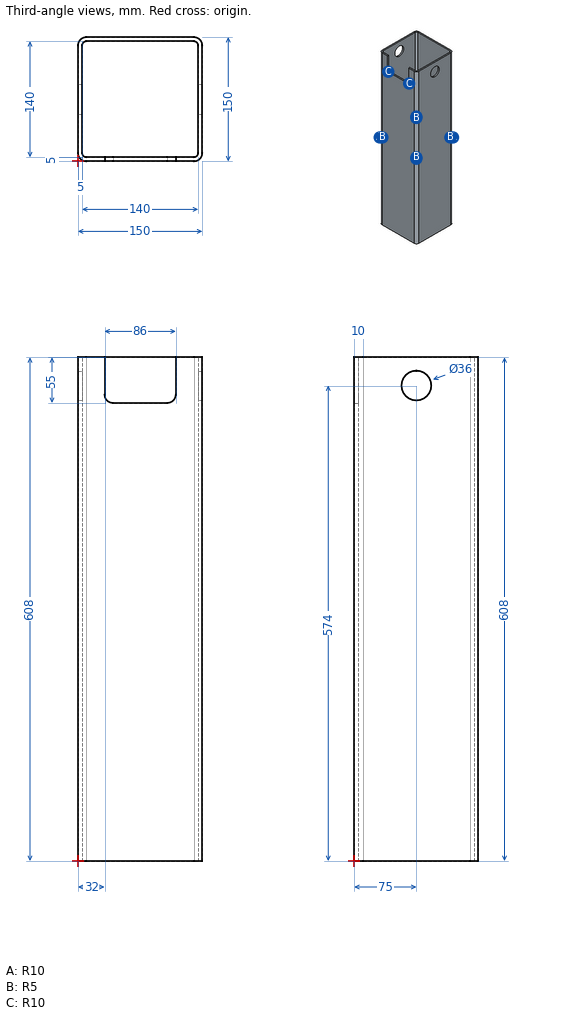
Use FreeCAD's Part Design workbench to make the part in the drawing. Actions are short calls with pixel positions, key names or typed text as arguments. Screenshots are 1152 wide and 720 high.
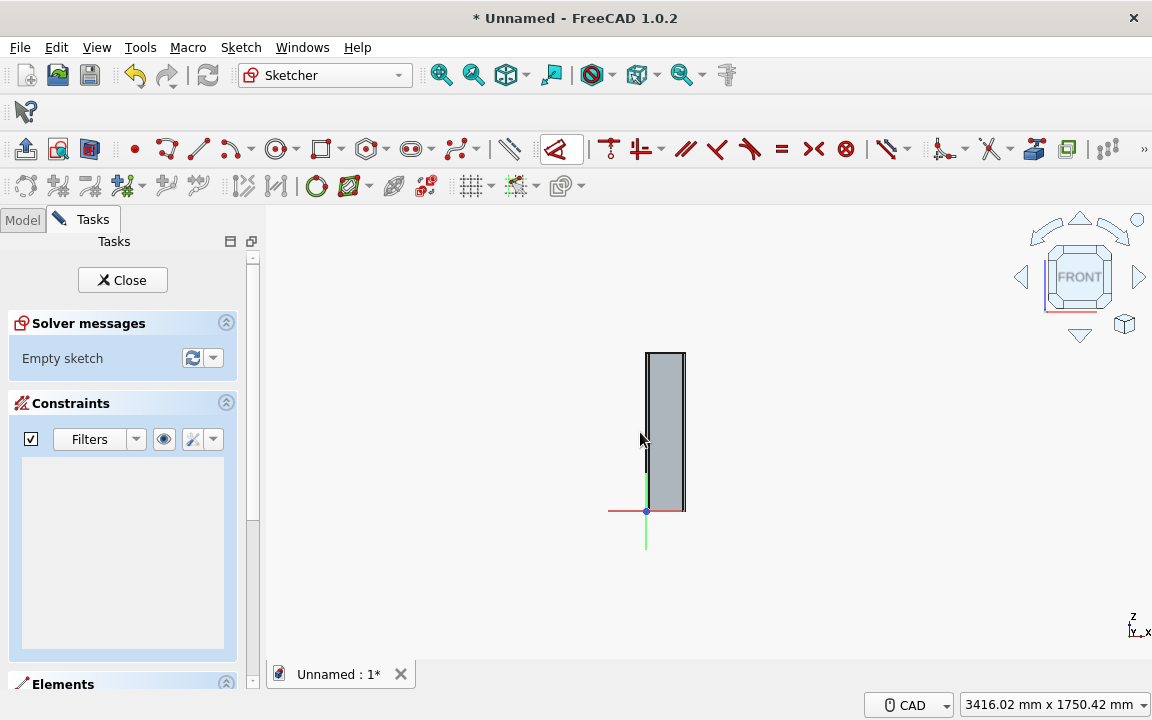
scroll(667, 357, up, 15)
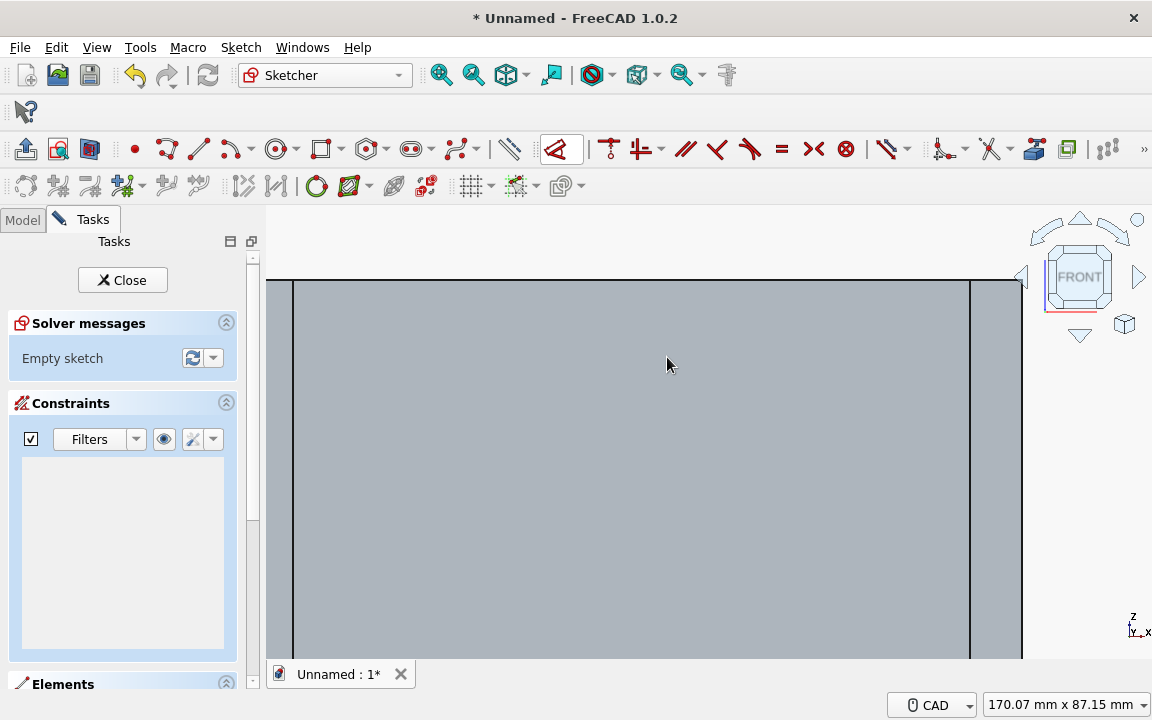
key(g)
key(r)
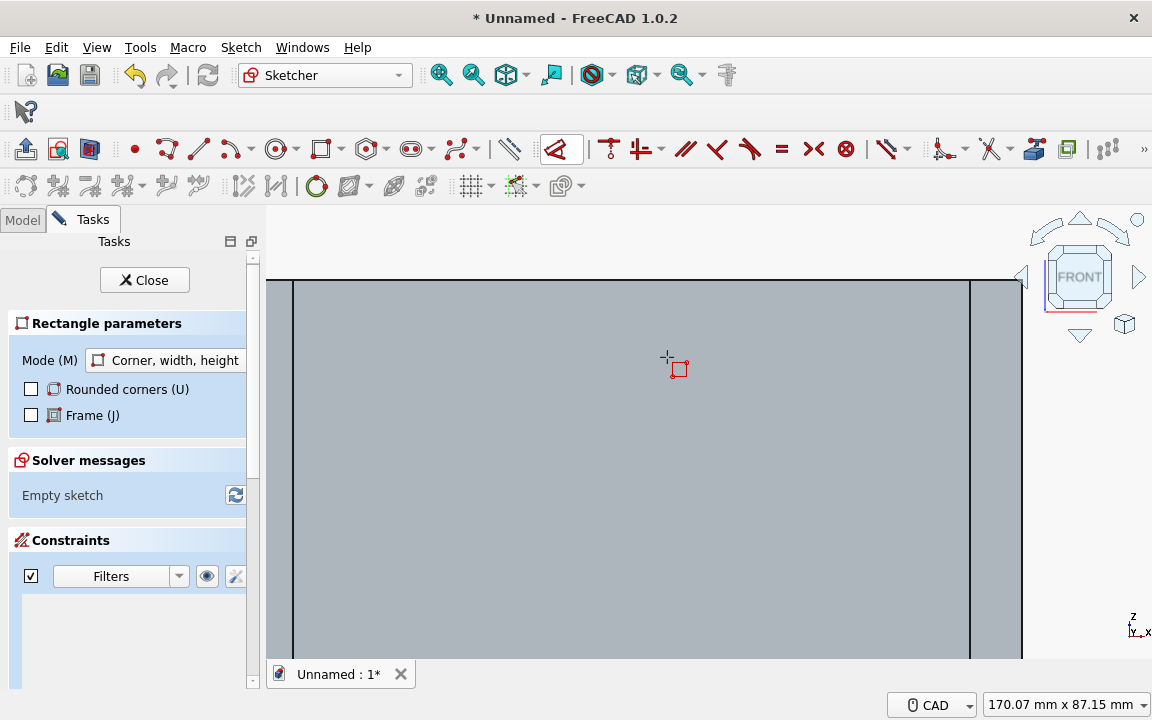
click(407, 280)
click(855, 566)
key(Escape)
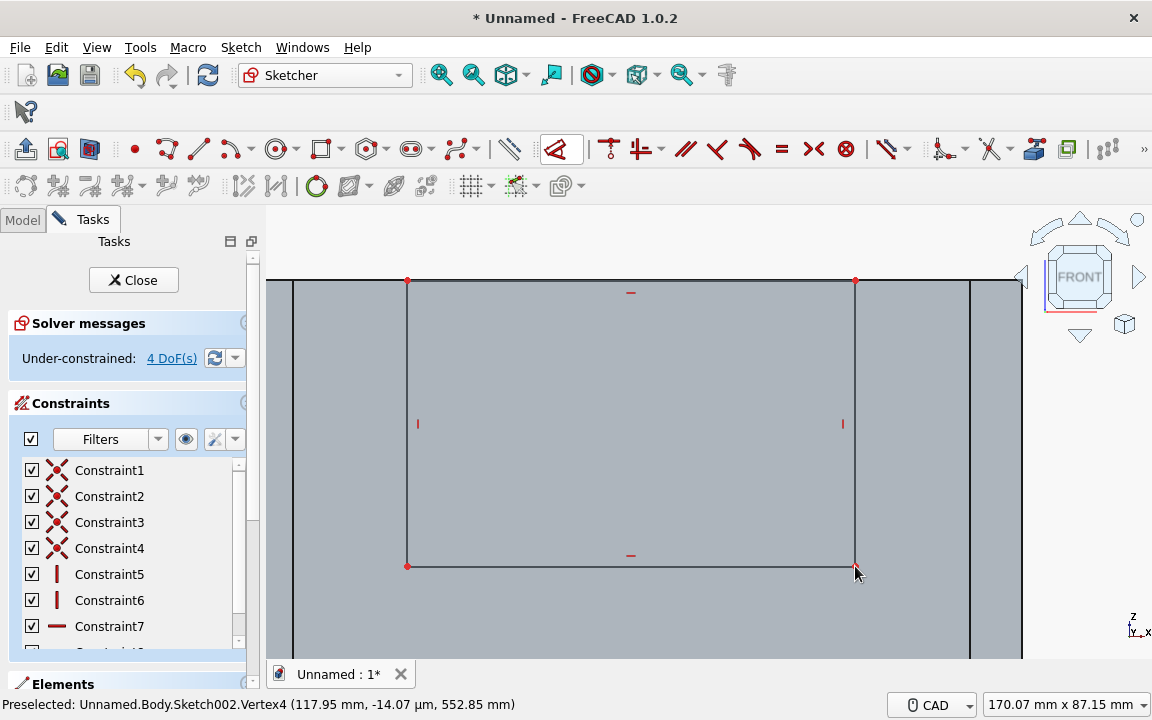
click(407, 367)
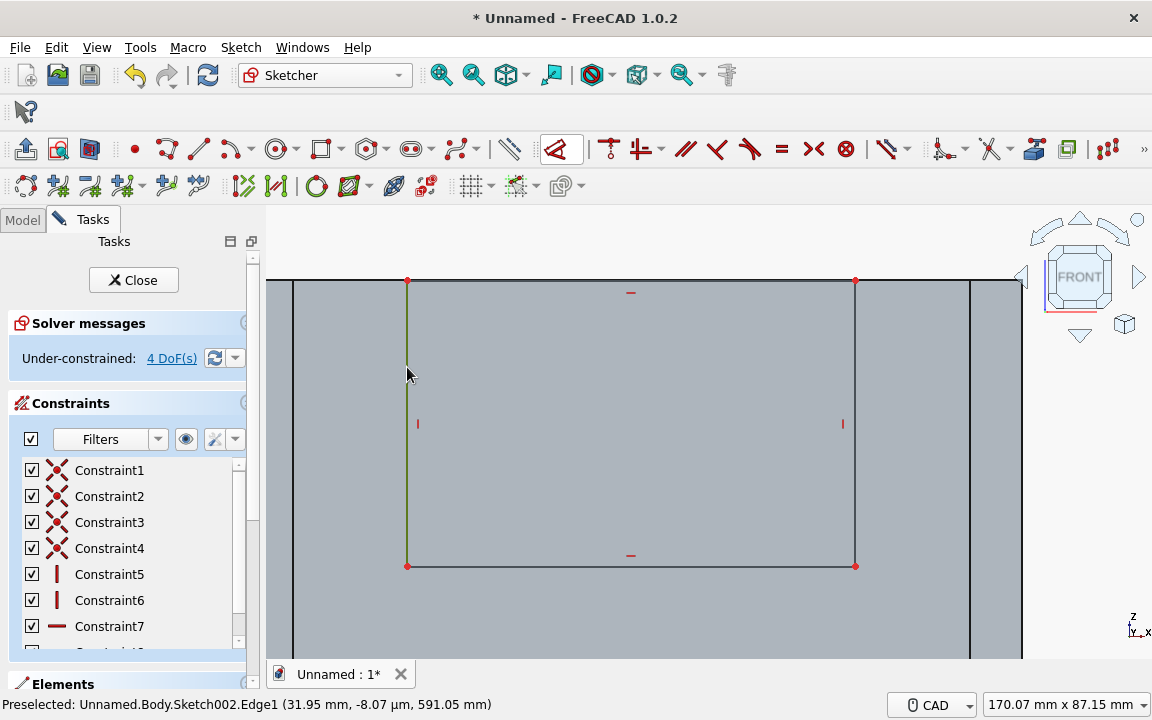
key(i)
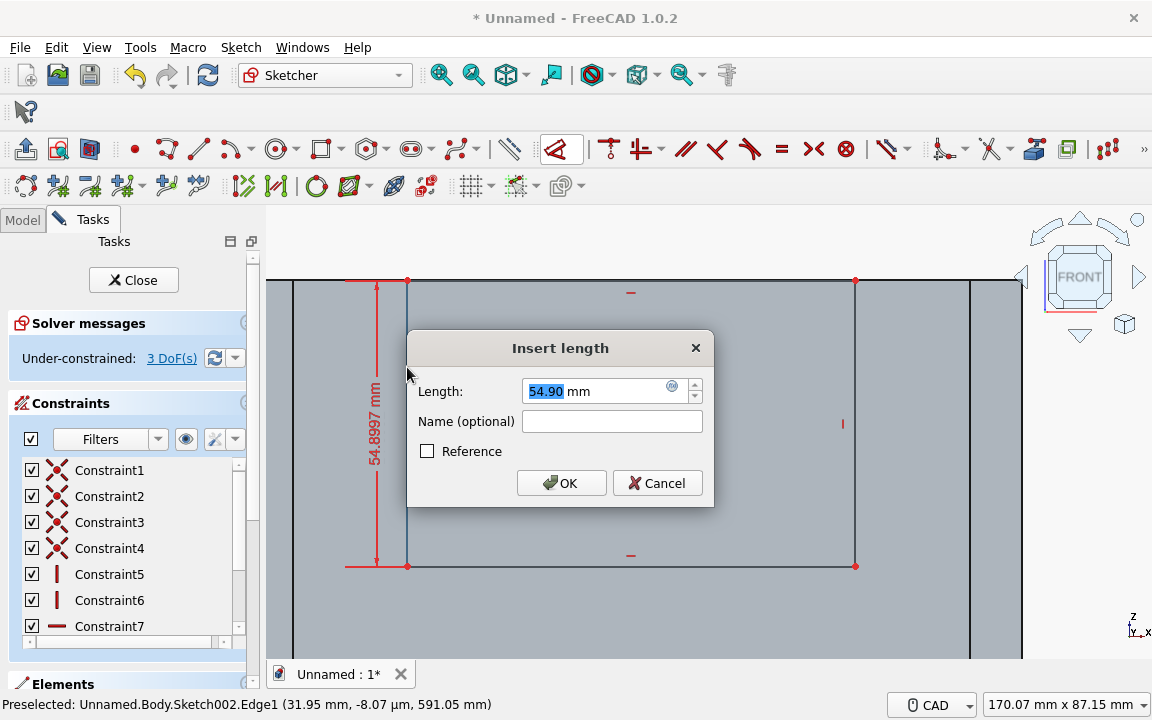
text(55)
key(Return)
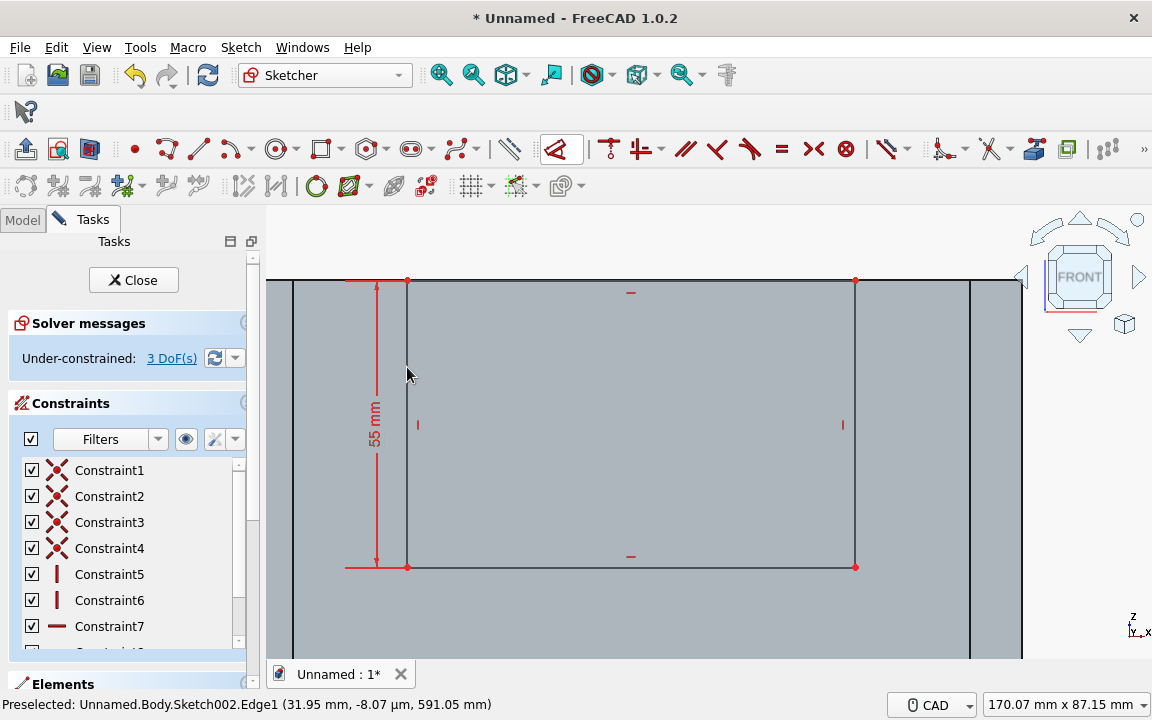
click(541, 568)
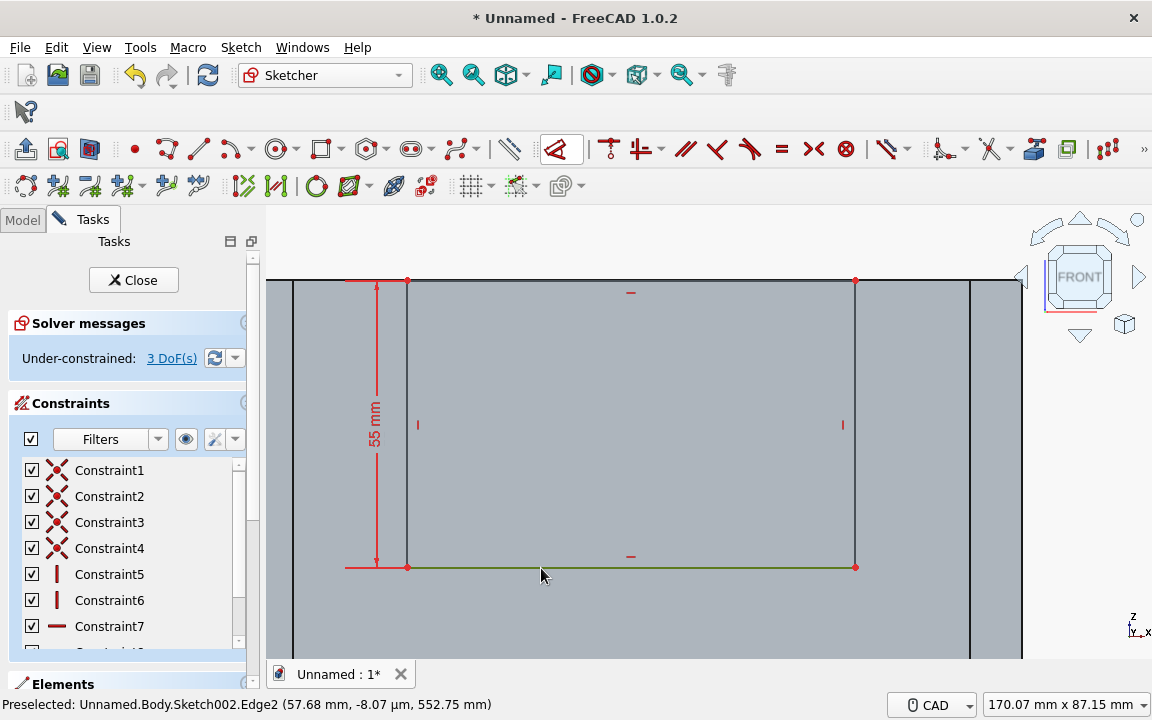
key(l)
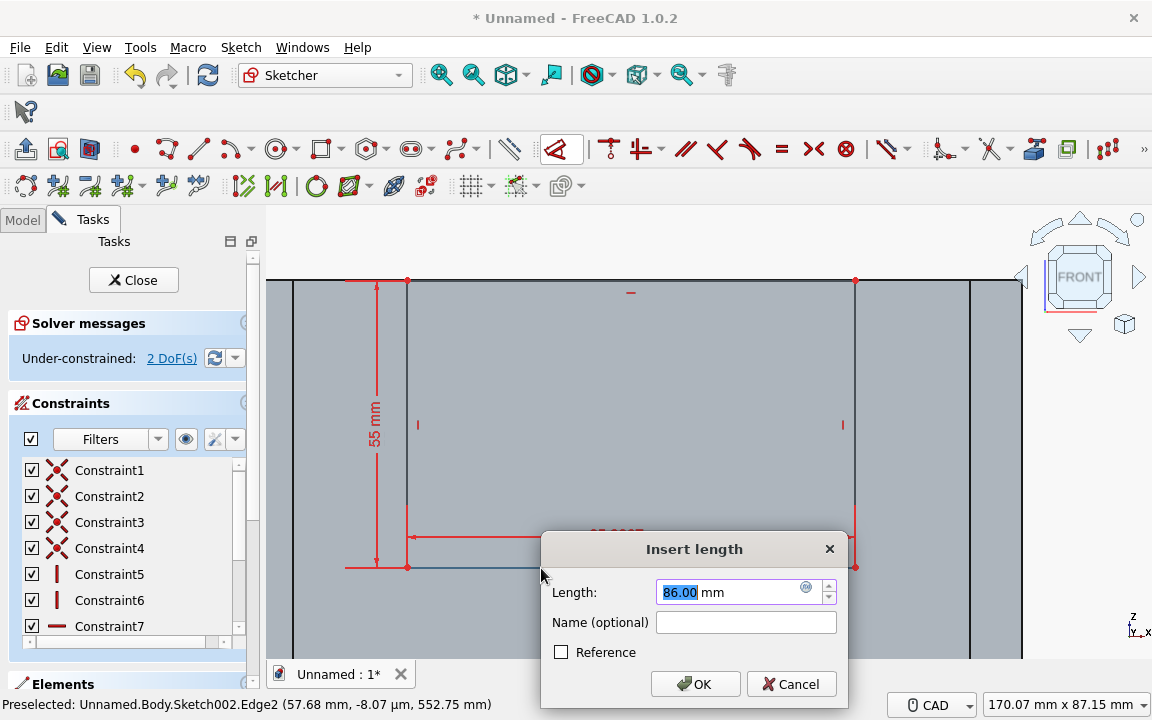
text(86)
key(Return)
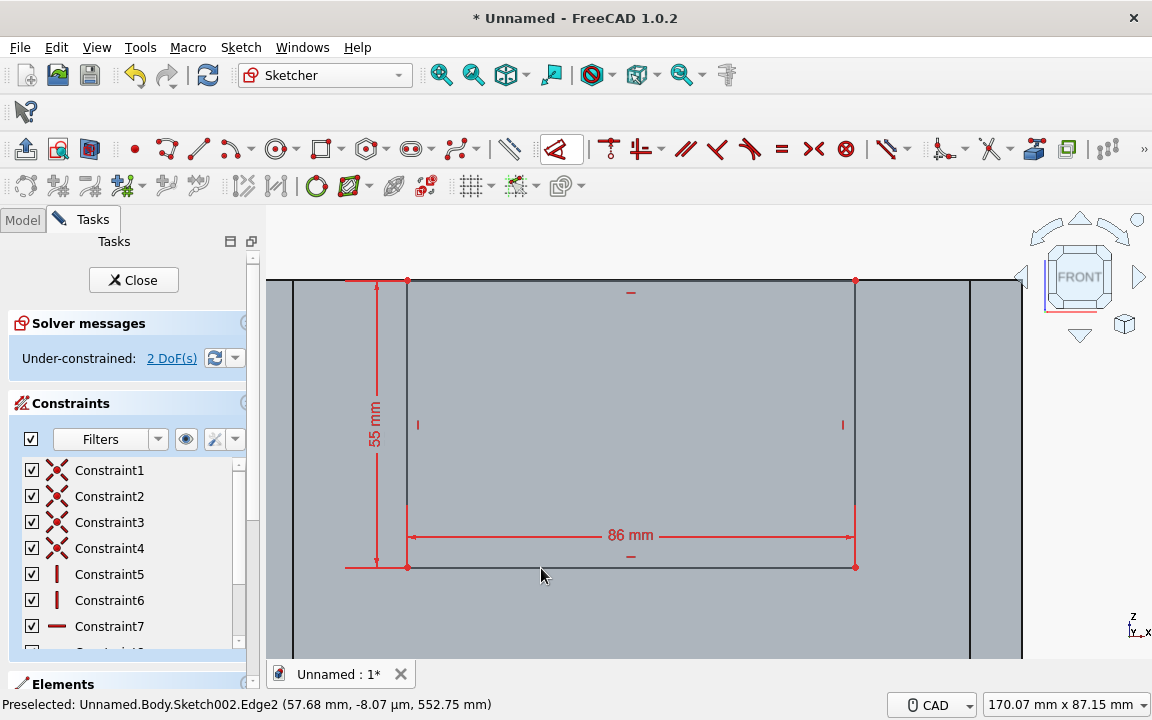
click(407, 281)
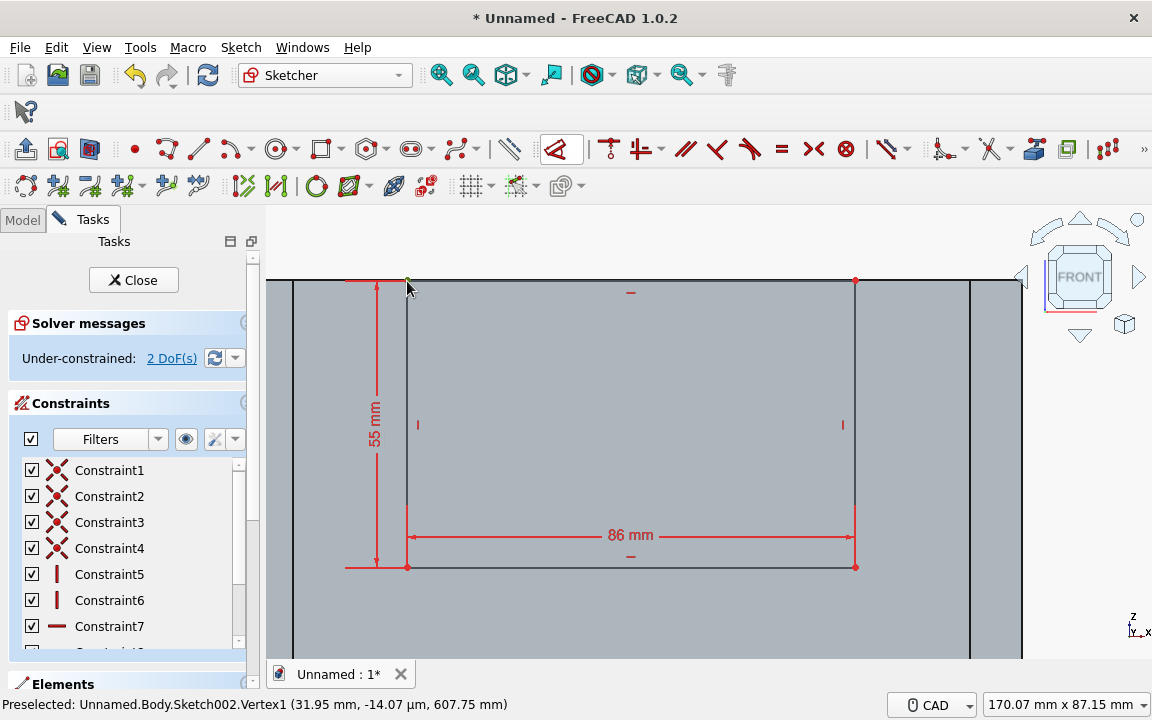
key(l)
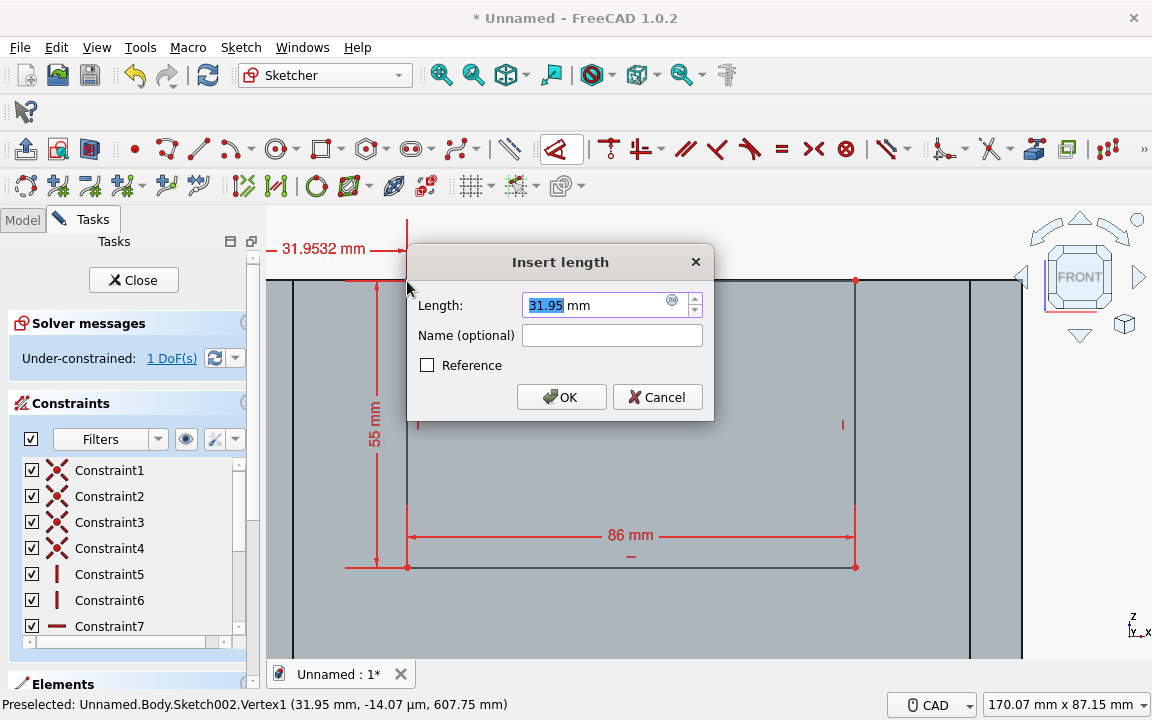
text(32)
key(Return)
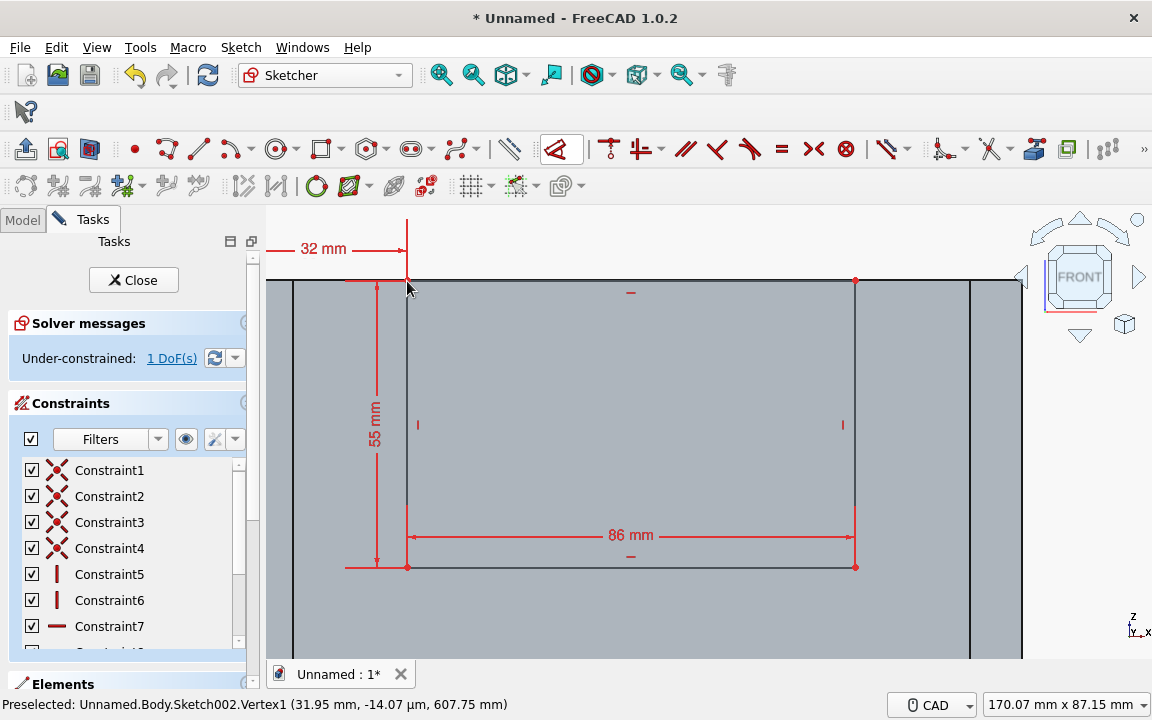
click(407, 281)